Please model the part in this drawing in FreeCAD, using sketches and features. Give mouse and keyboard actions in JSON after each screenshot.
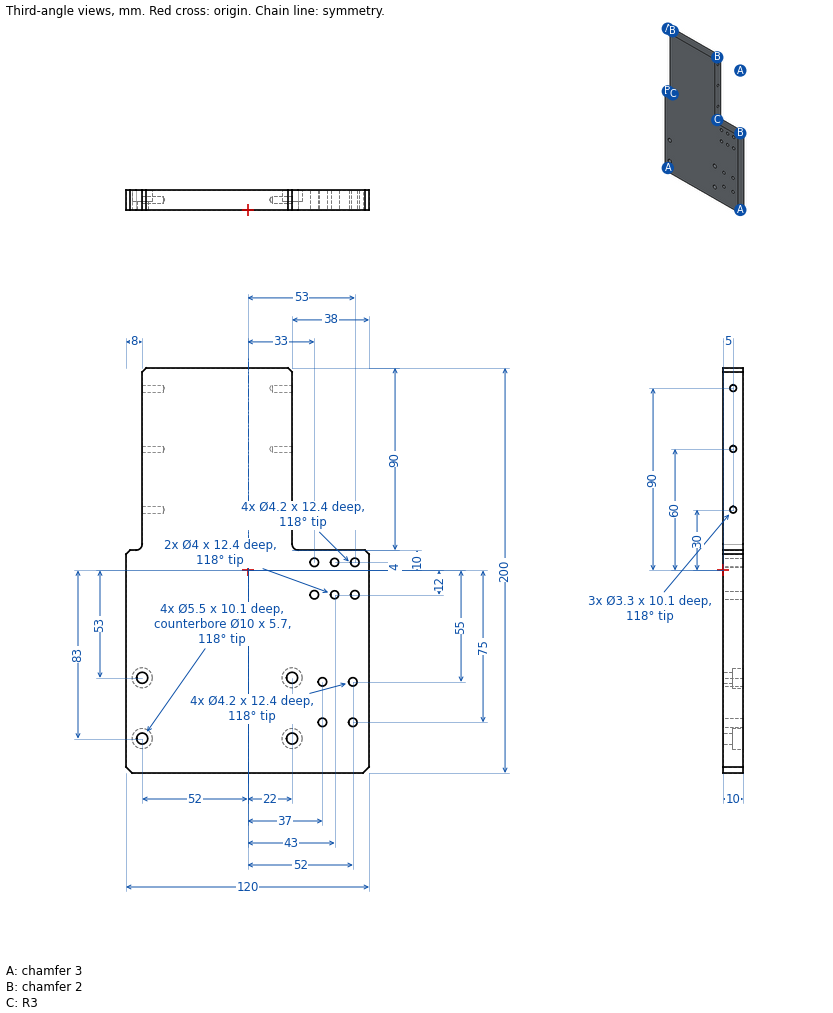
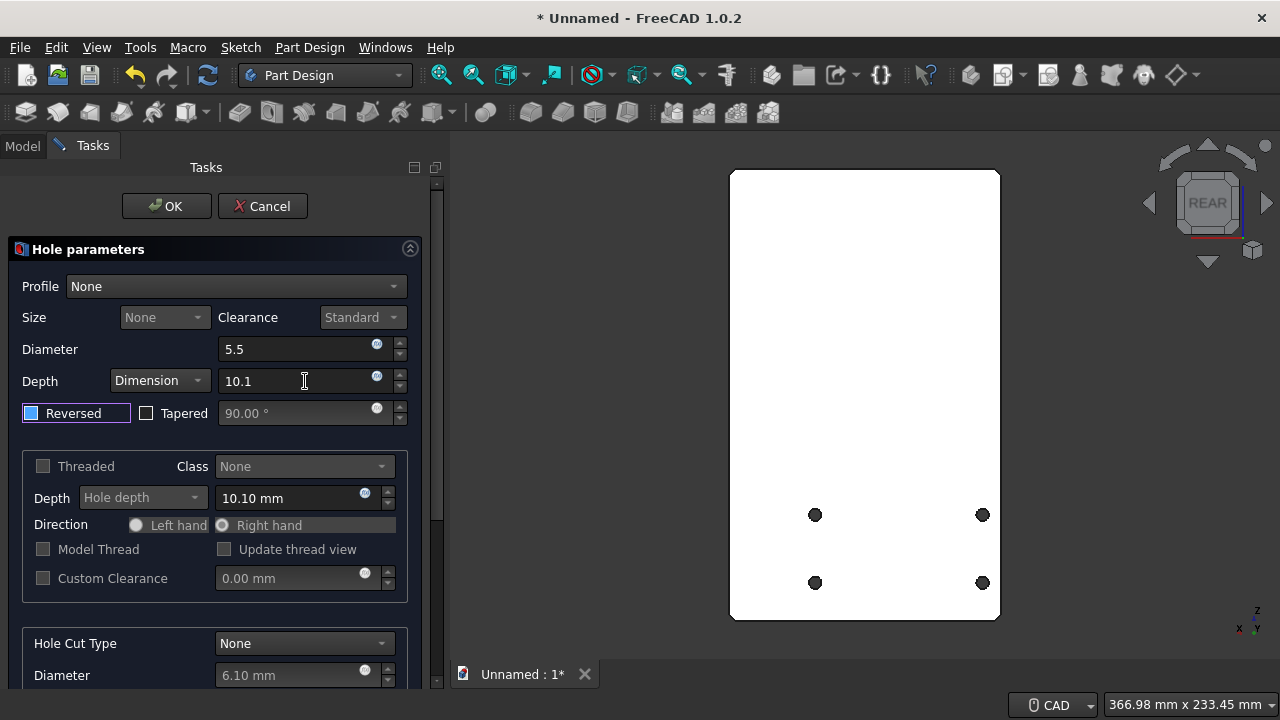
{"action": "left_click", "coordinate": [306, 644]}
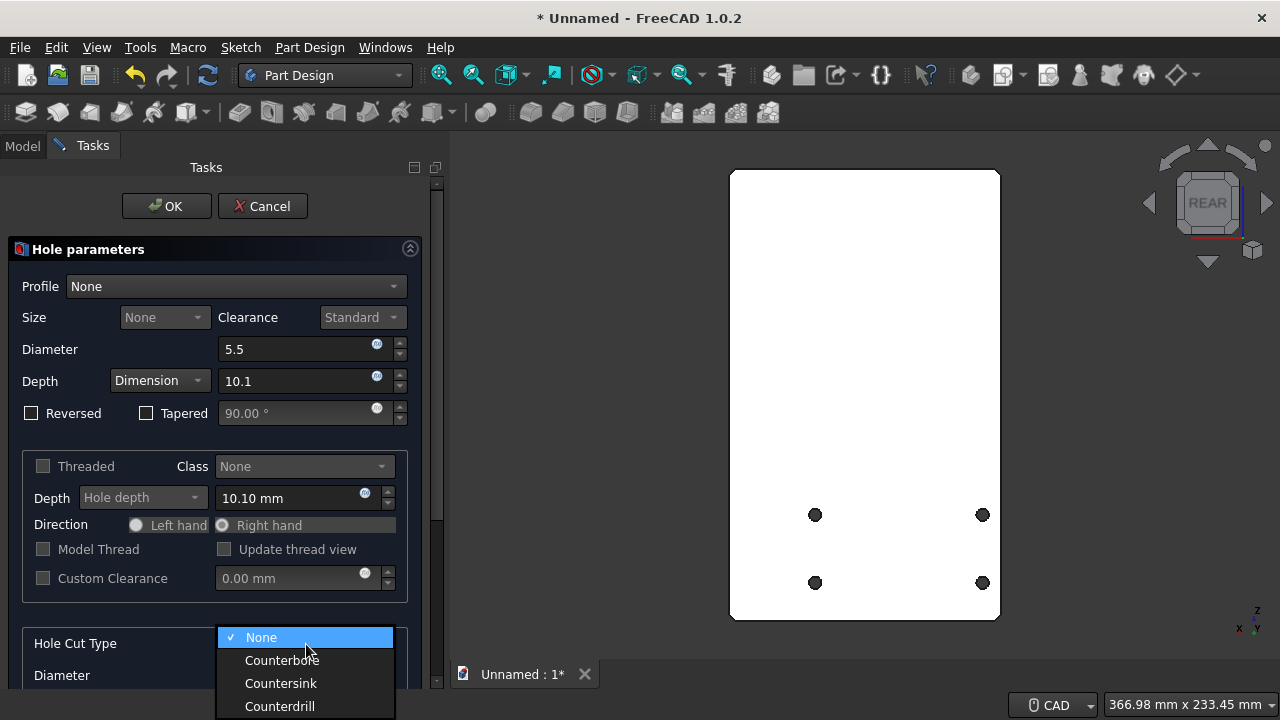
{"action": "left_click", "coordinate": [304, 660]}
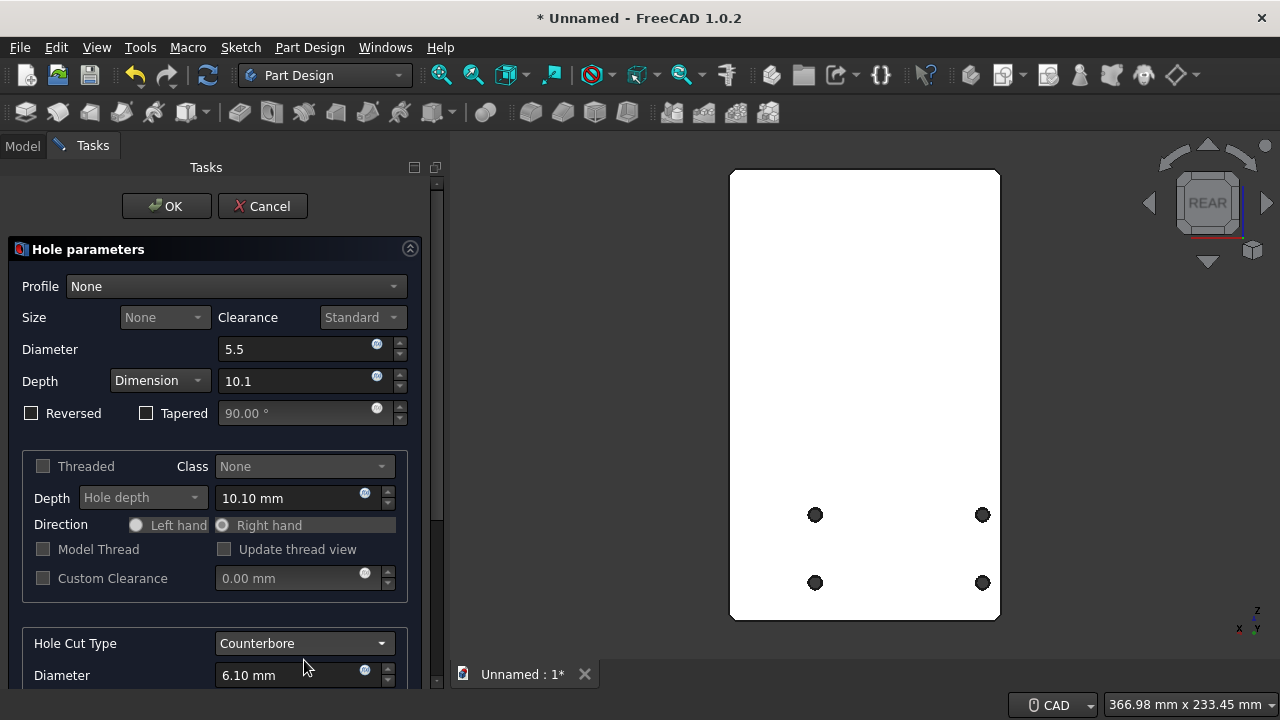
{"action": "triple_click", "coordinate": [298, 675]}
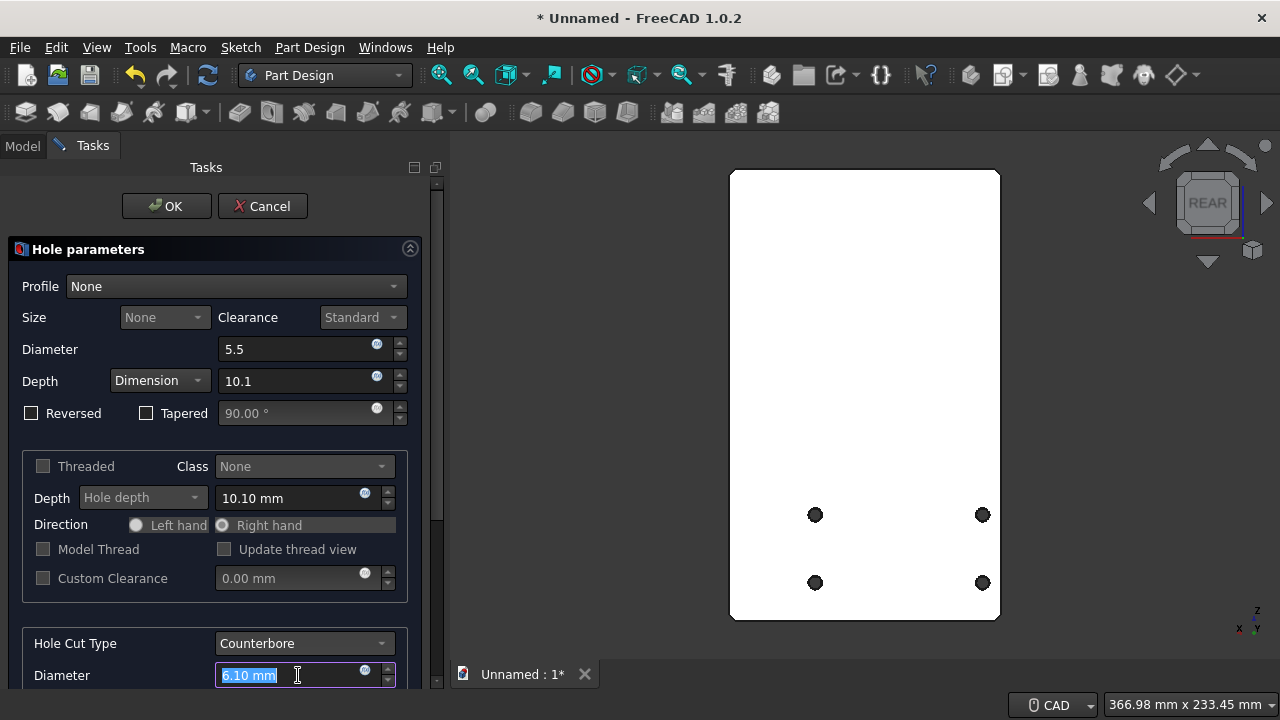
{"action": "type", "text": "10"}
{"action": "key", "text": "Tab"}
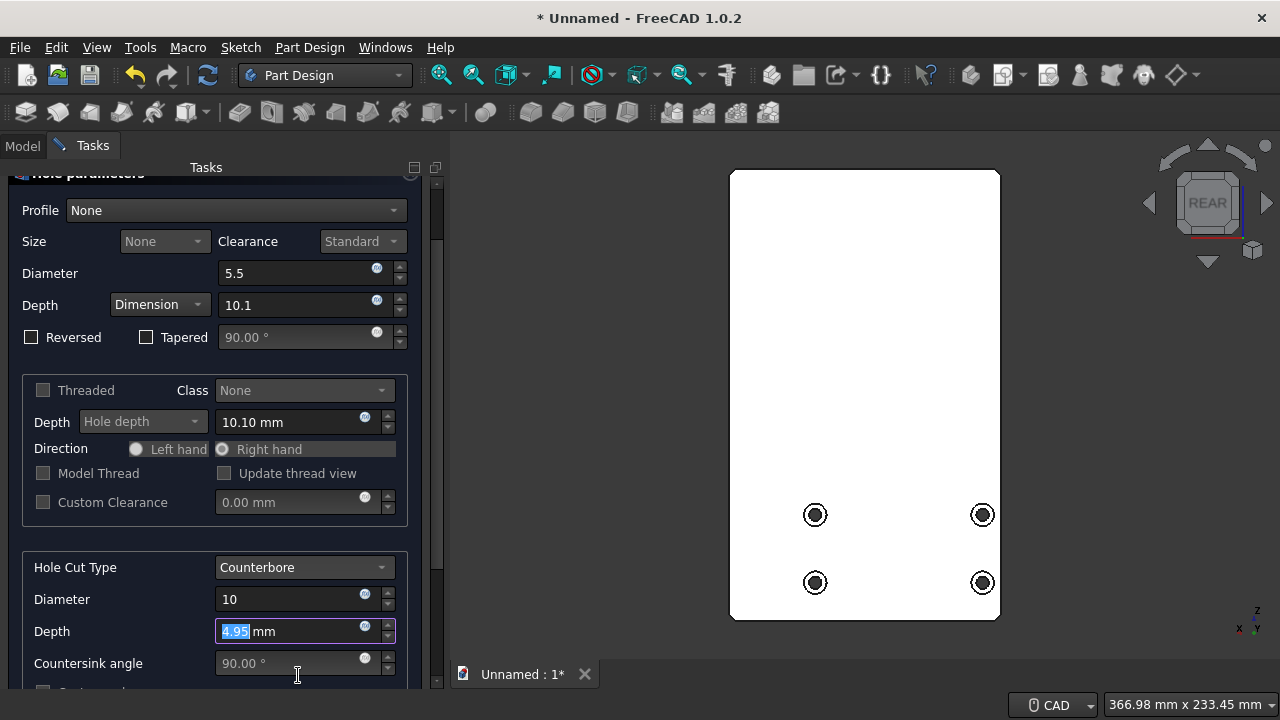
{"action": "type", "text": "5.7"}
{"action": "key", "text": "Tab"}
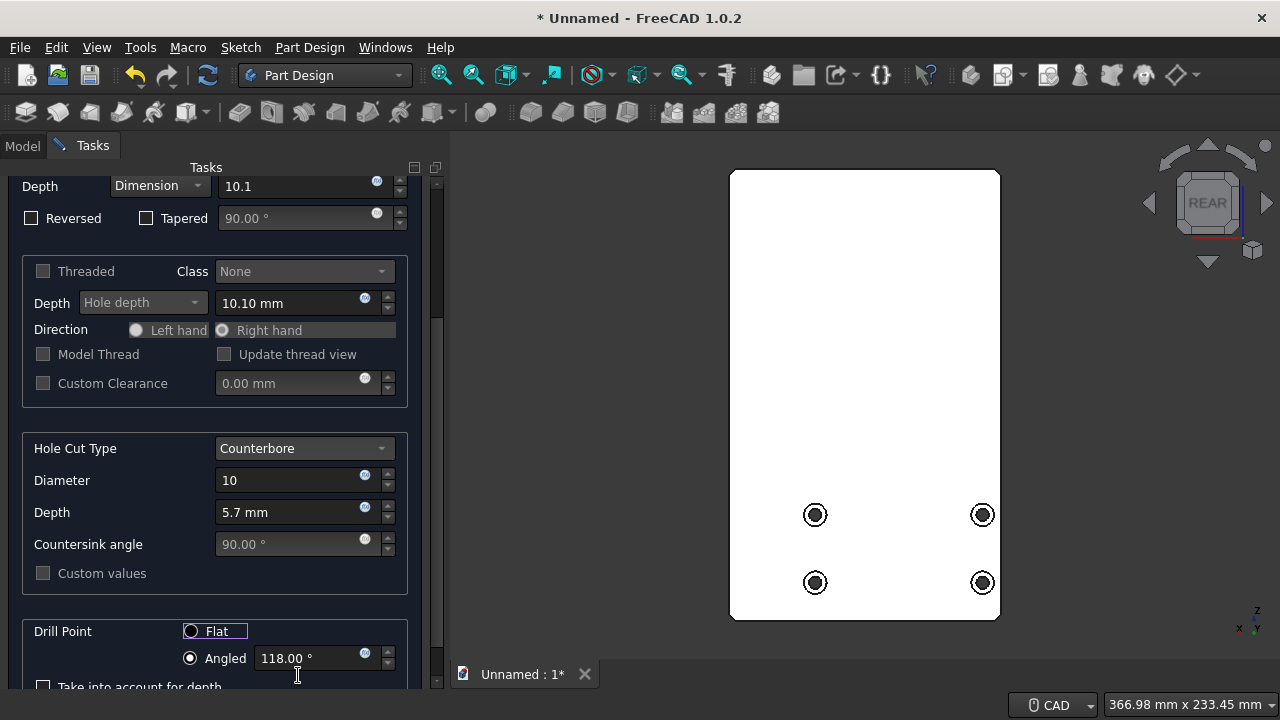
{"action": "scroll", "coordinate": [437, 432], "scroll_direction": "up", "scroll_amount": 4}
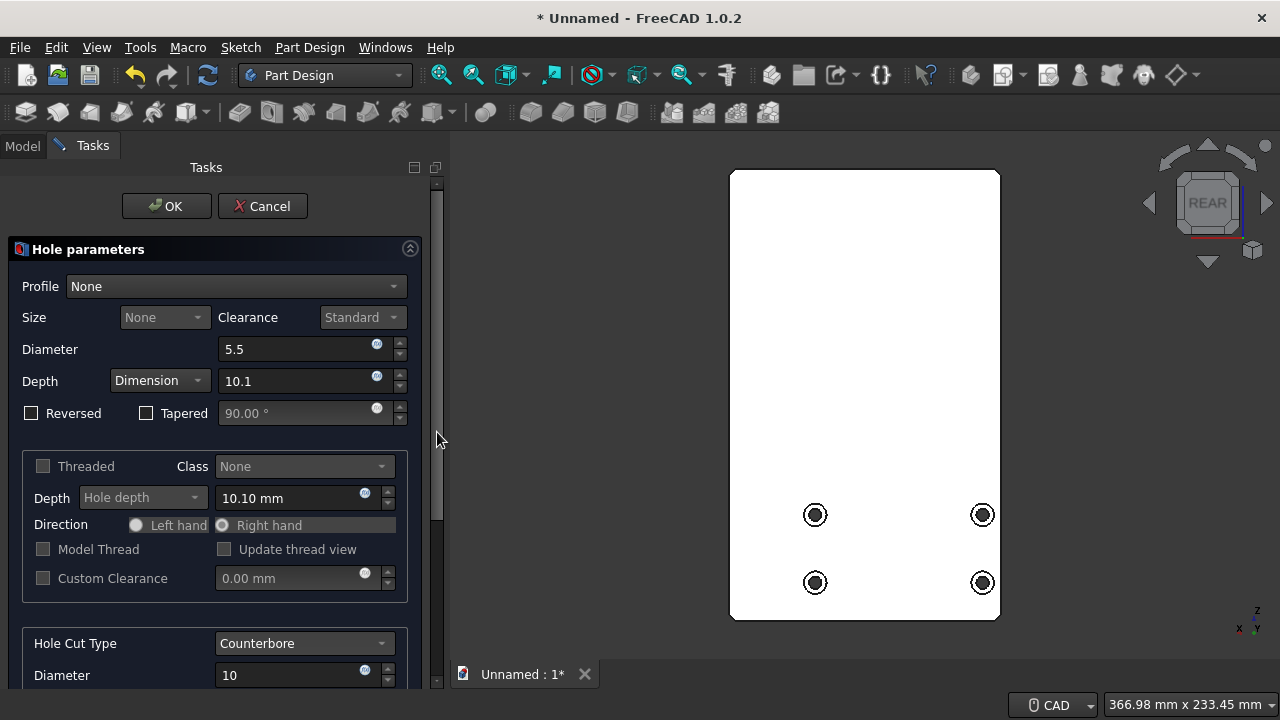
{"action": "left_click", "coordinate": [167, 206]}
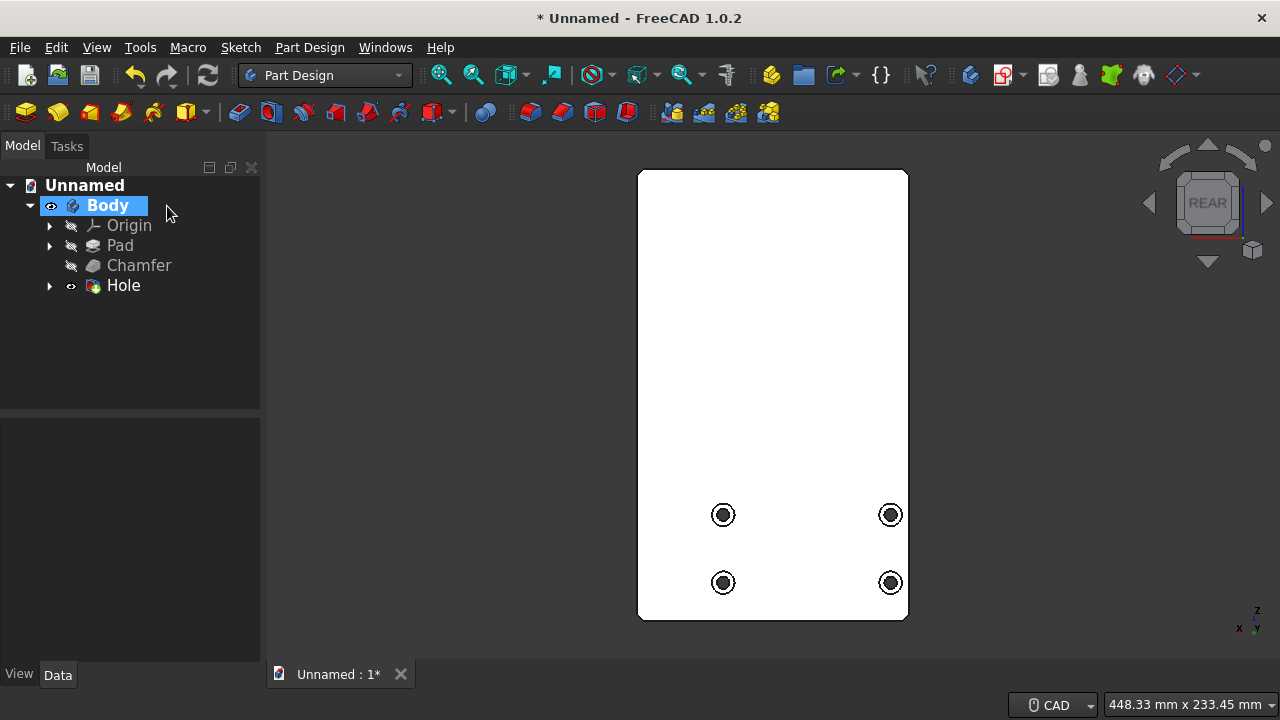
{"action": "left_click", "coordinate": [773, 329]}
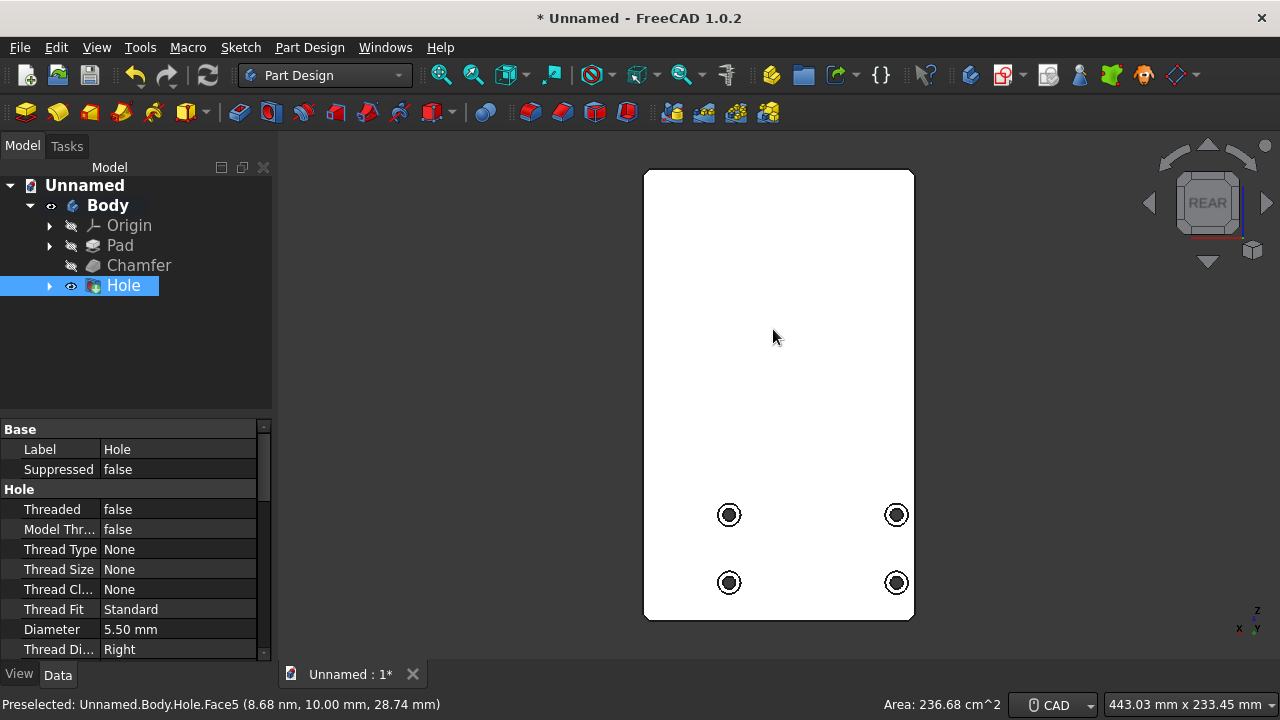
{"action": "left_click", "coordinate": [1004, 76]}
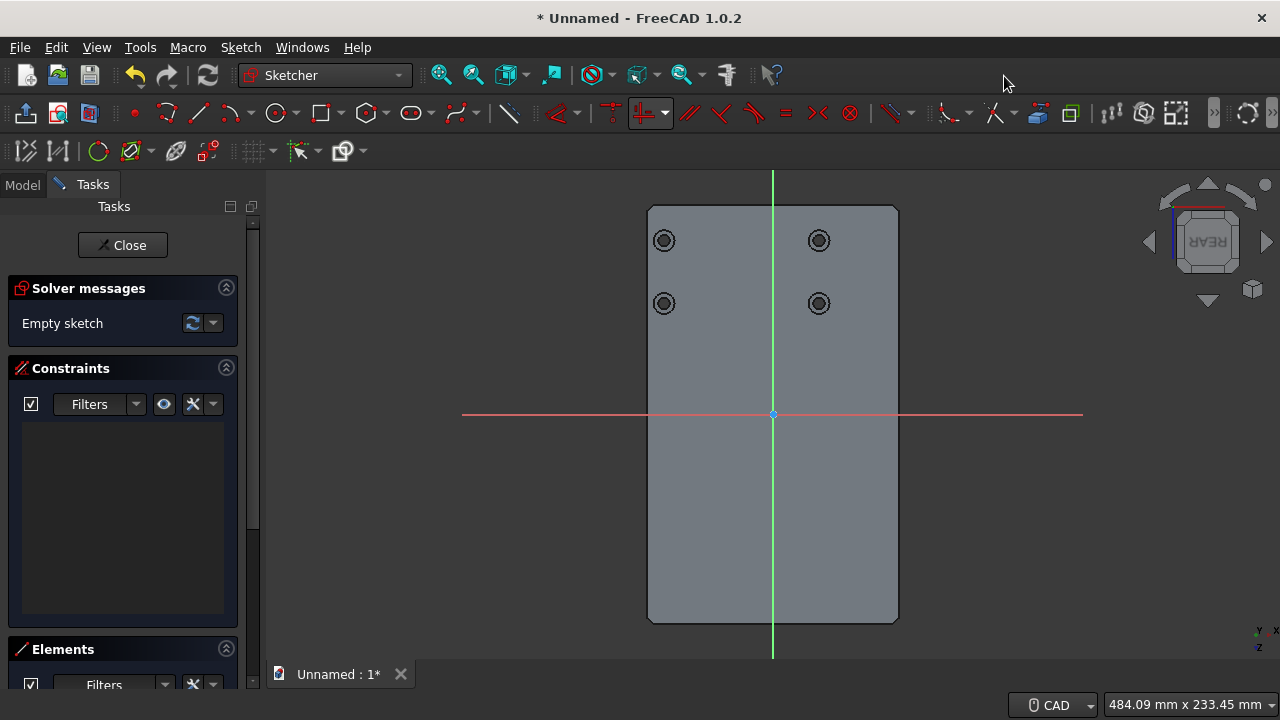
{"action": "scroll", "coordinate": [395, 198], "scroll_direction": "down", "scroll_amount": 1}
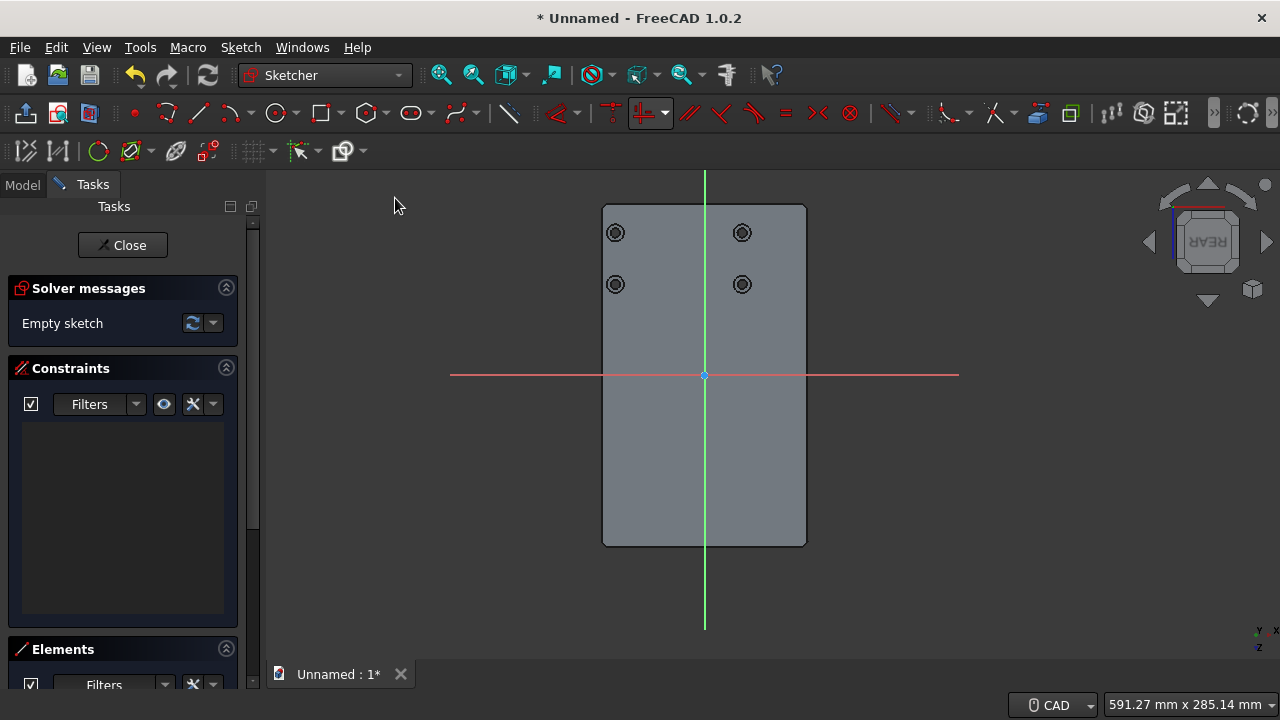
{"action": "scroll", "coordinate": [705, 518], "scroll_direction": "up", "scroll_amount": 3}